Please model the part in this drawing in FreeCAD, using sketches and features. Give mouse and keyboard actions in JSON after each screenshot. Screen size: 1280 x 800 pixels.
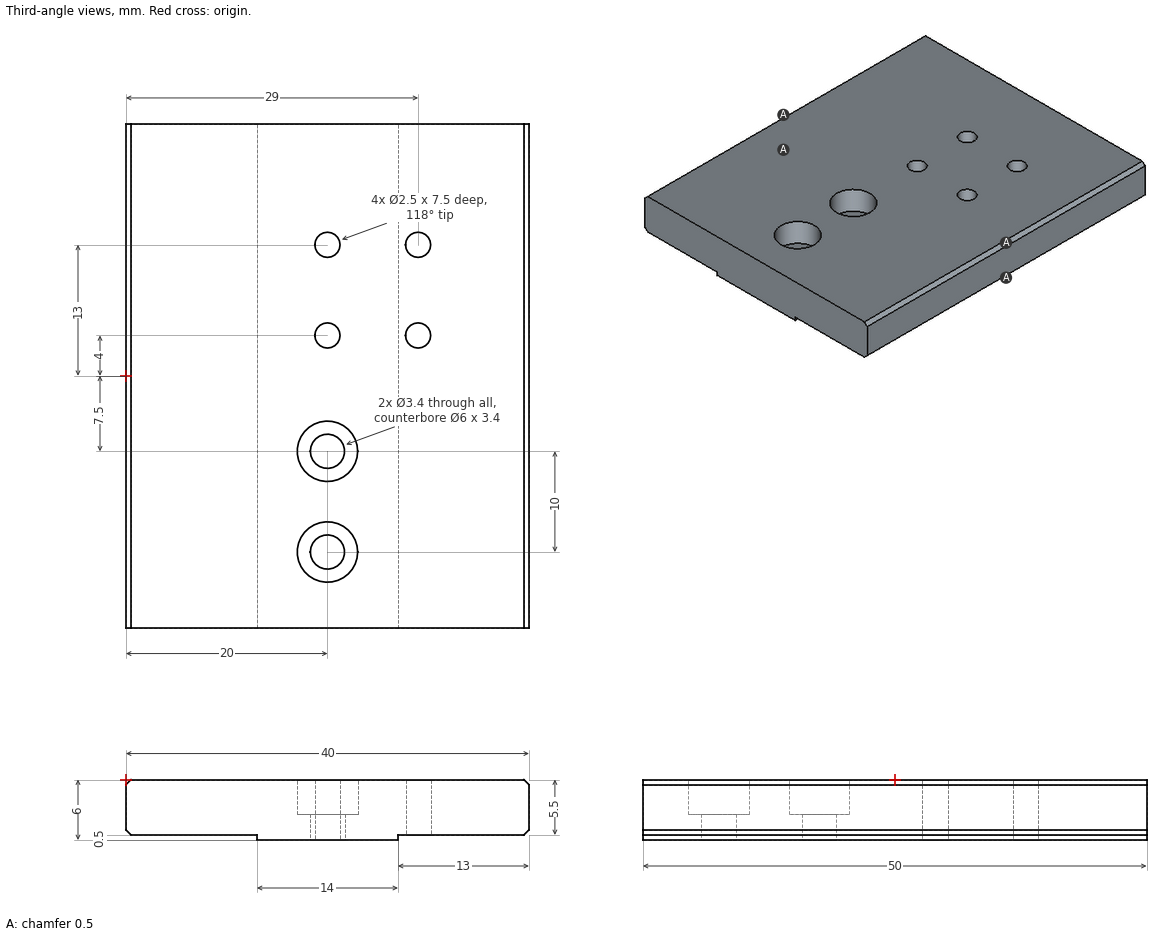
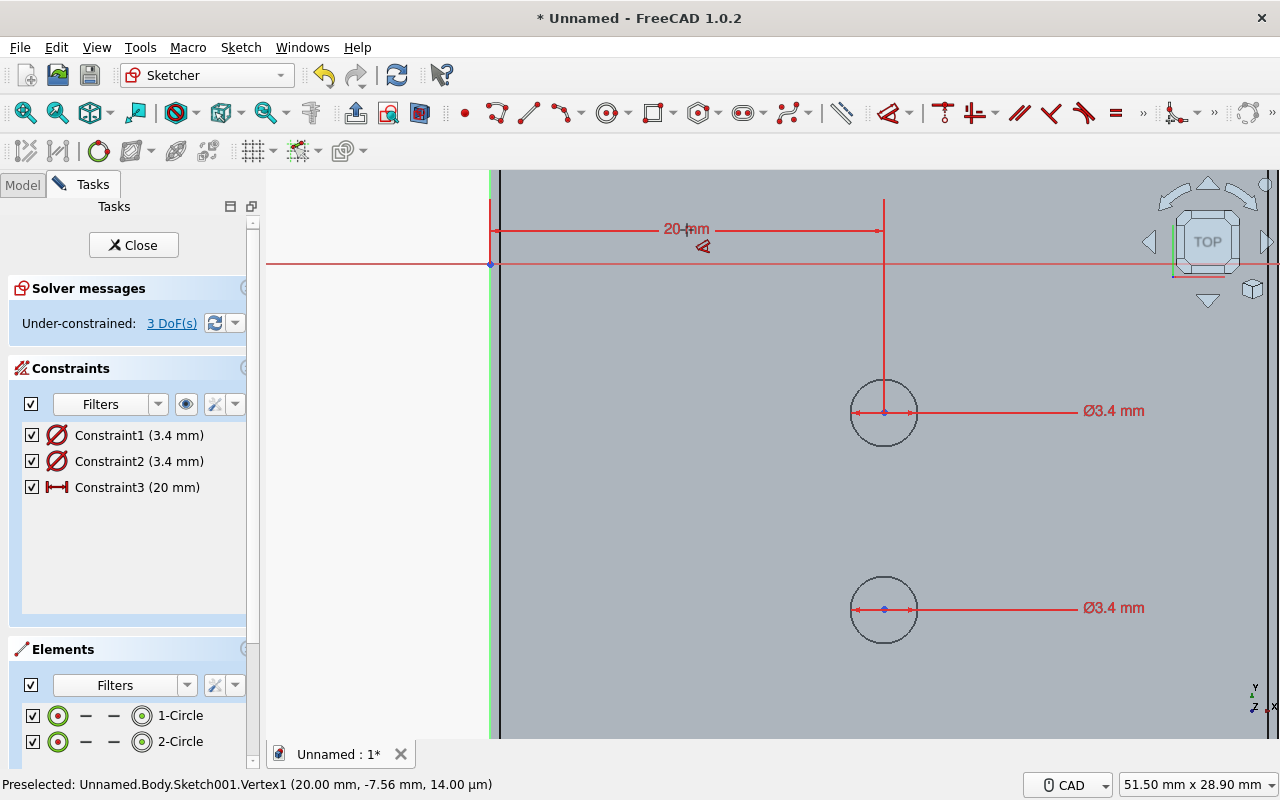
{"action": "left_click", "coordinate": [884, 610]}
{"action": "left_click", "coordinate": [597, 230]}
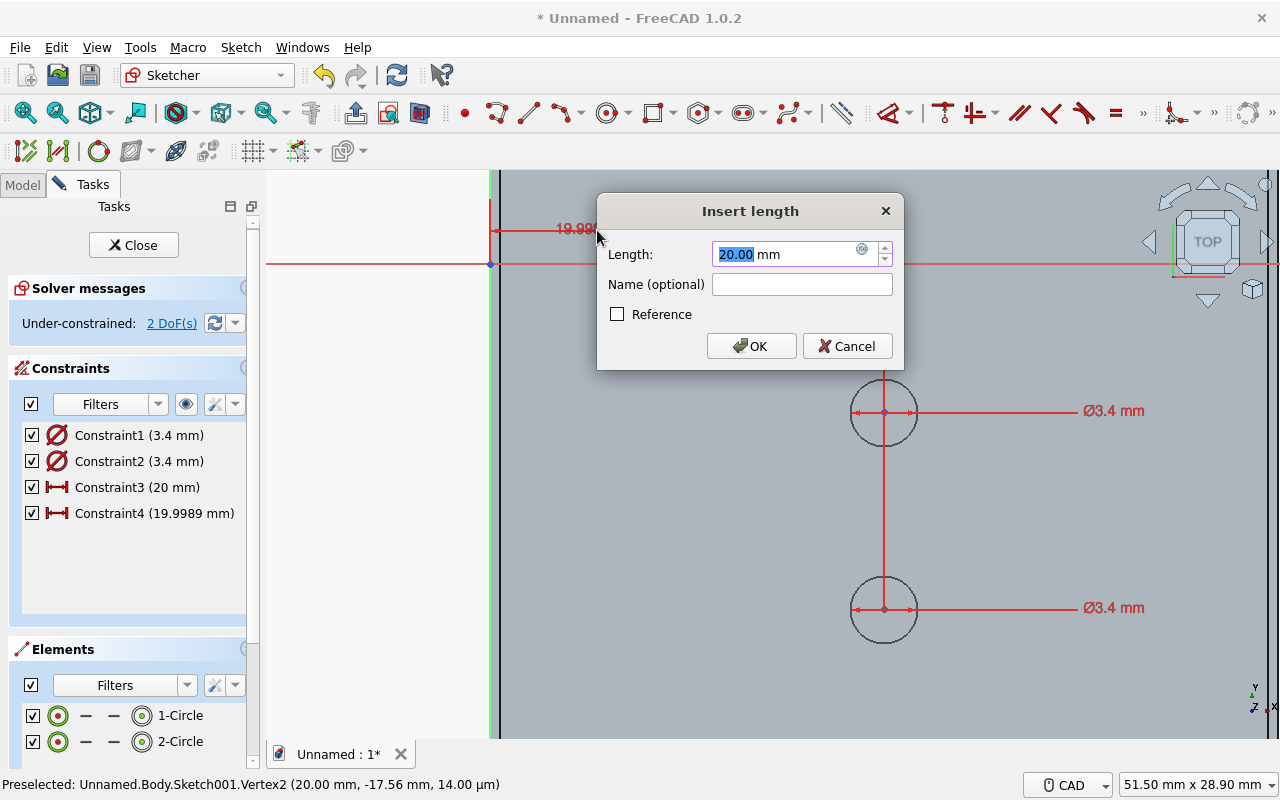
{"action": "type", "text": "20"}
{"action": "key", "text": "Return"}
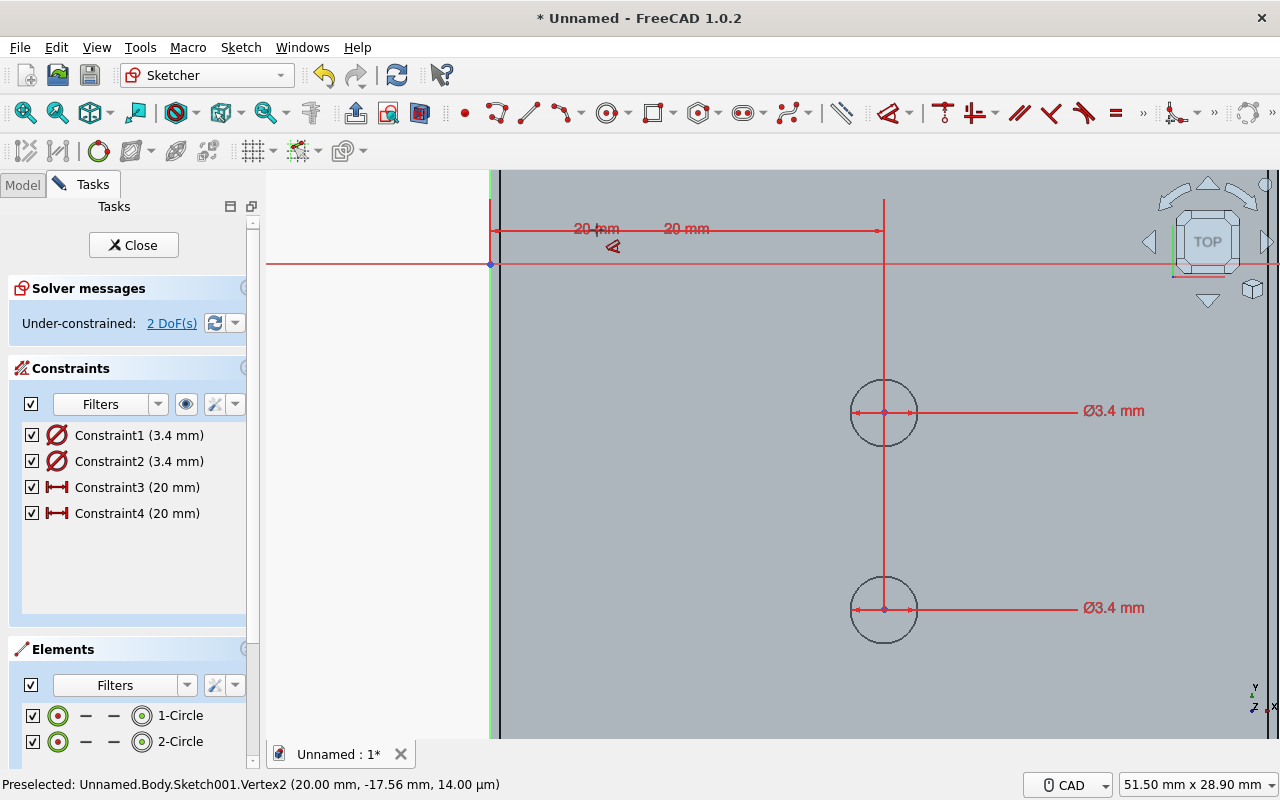
{"action": "left_click", "coordinate": [884, 413]}
{"action": "left_click", "coordinate": [456, 339]}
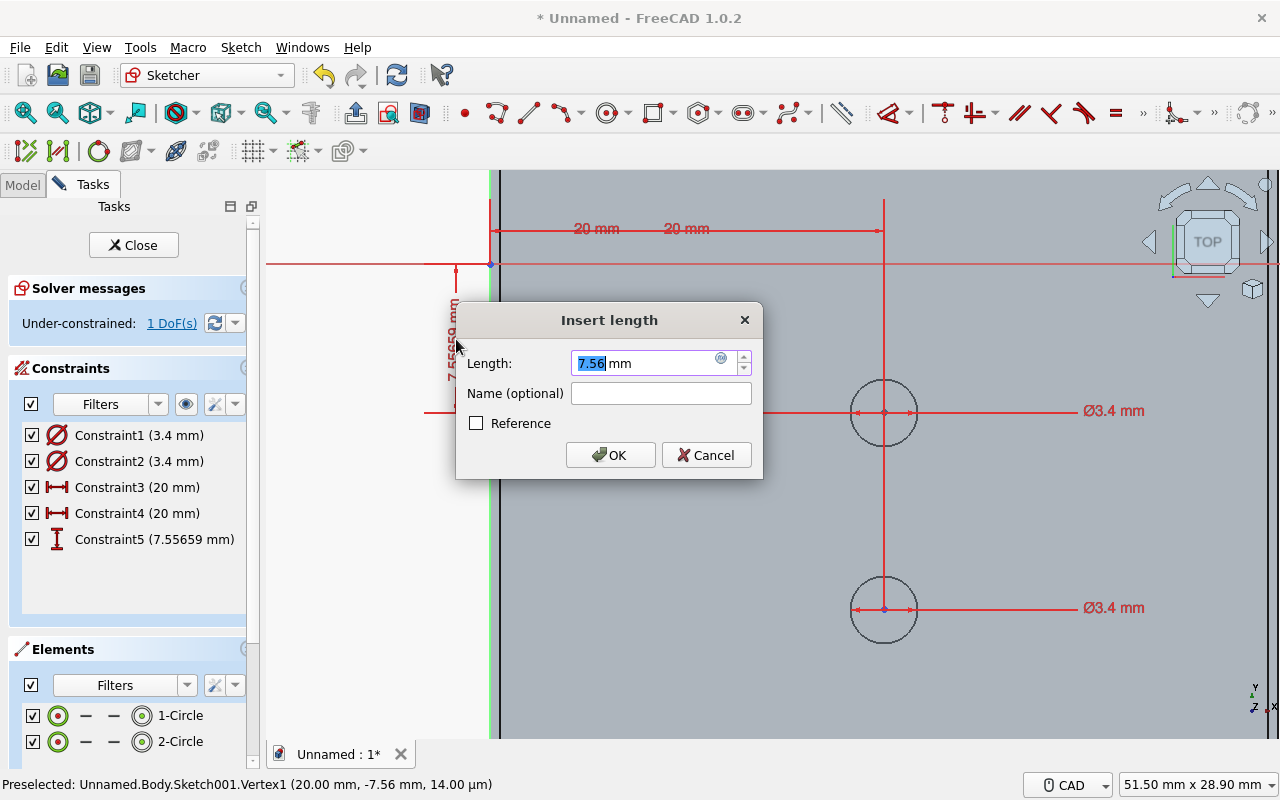
{"action": "type", "text": "7.5"}
{"action": "key", "text": "Return"}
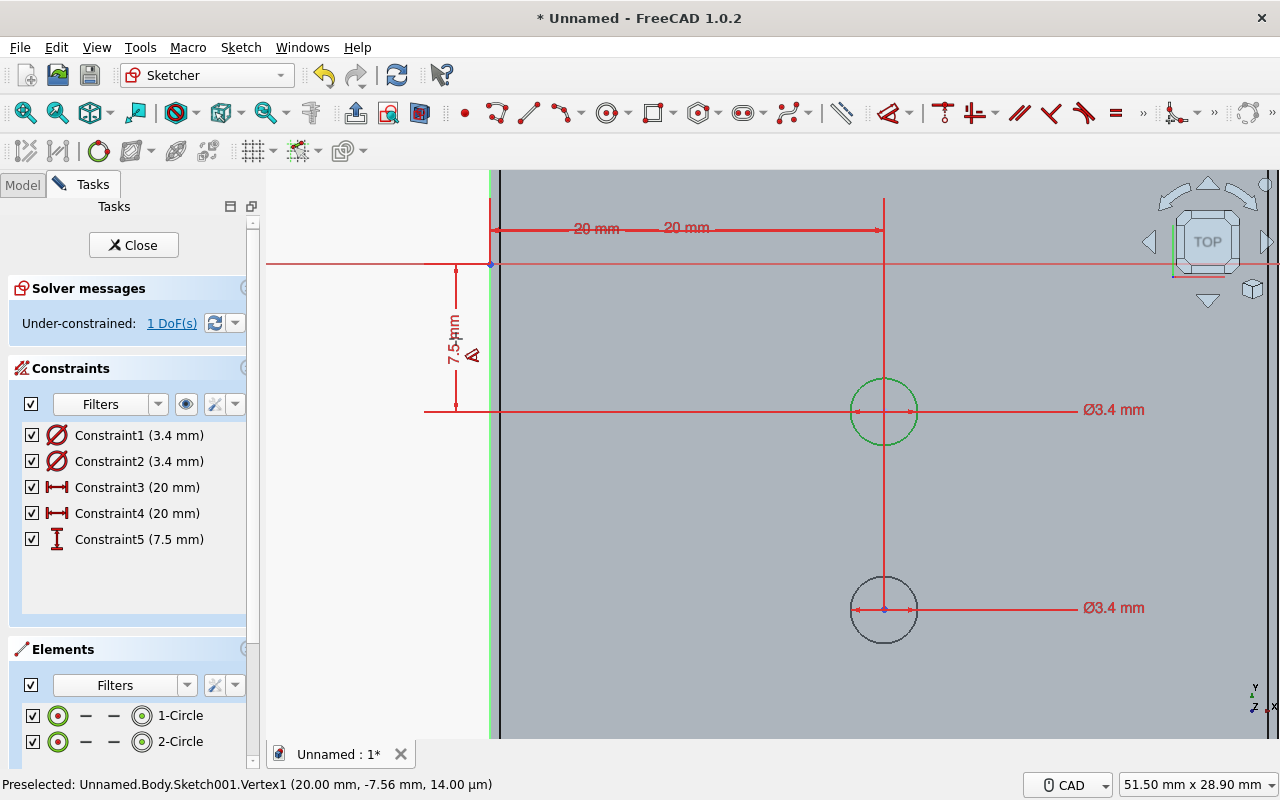
{"action": "left_click", "coordinate": [884, 412]}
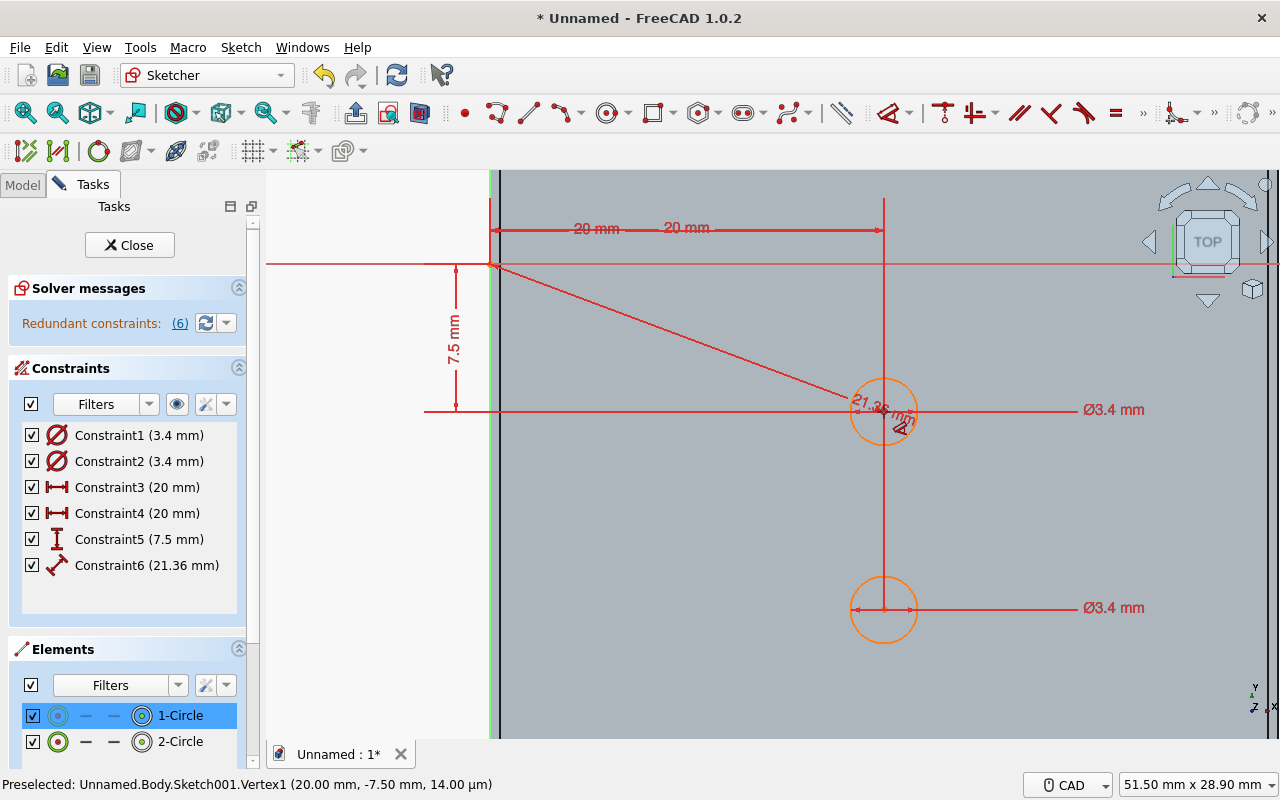
{"action": "left_click", "coordinate": [884, 610]}
{"action": "left_click", "coordinate": [918, 511]}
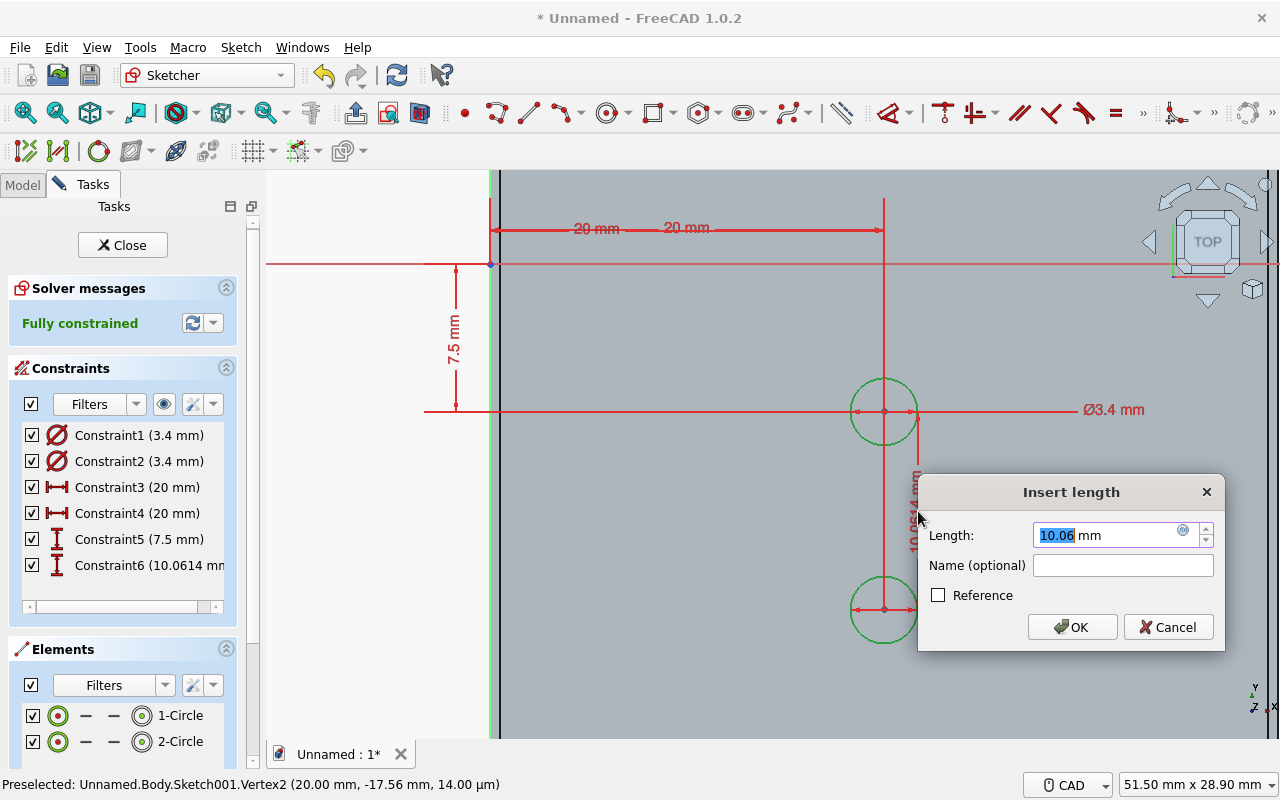
{"action": "type", "text": "10"}
{"action": "key", "text": "Return"}
{"action": "key", "text": "Escape"}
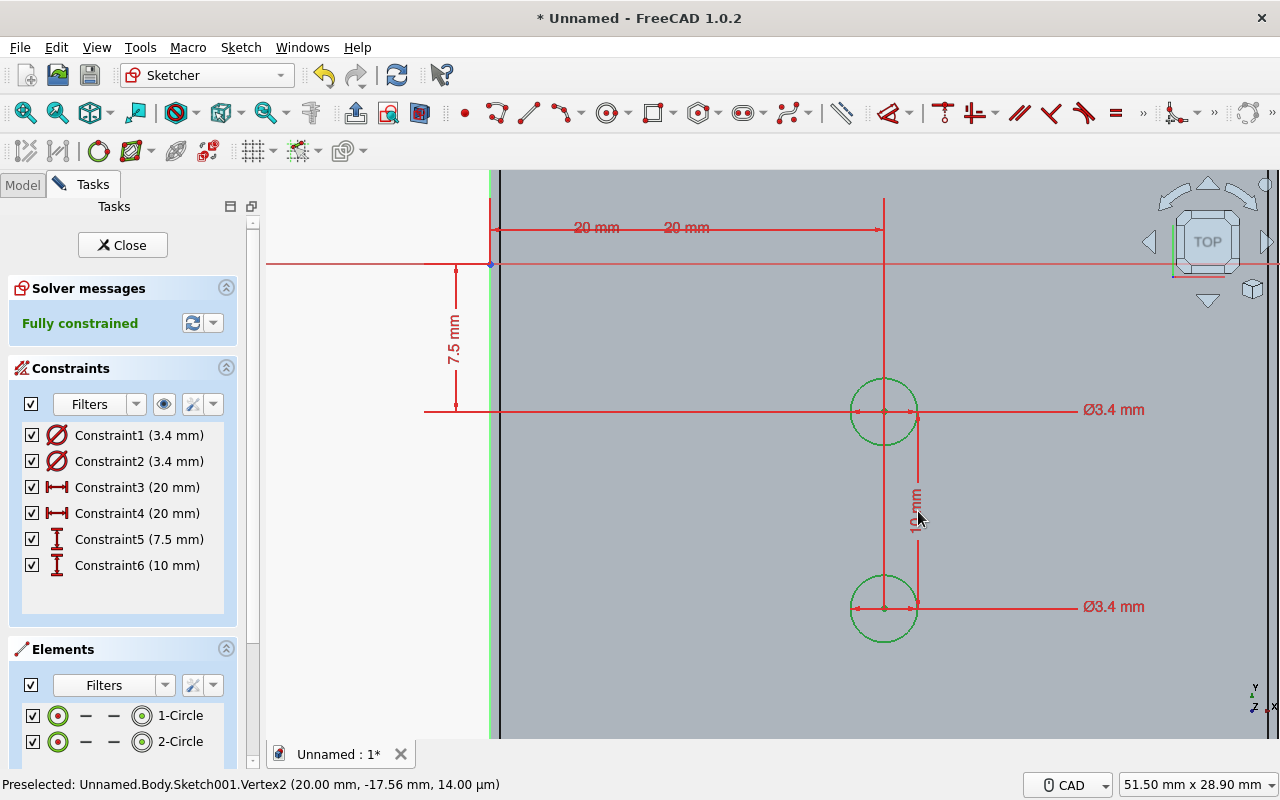
{"action": "left_click", "coordinate": [123, 245]}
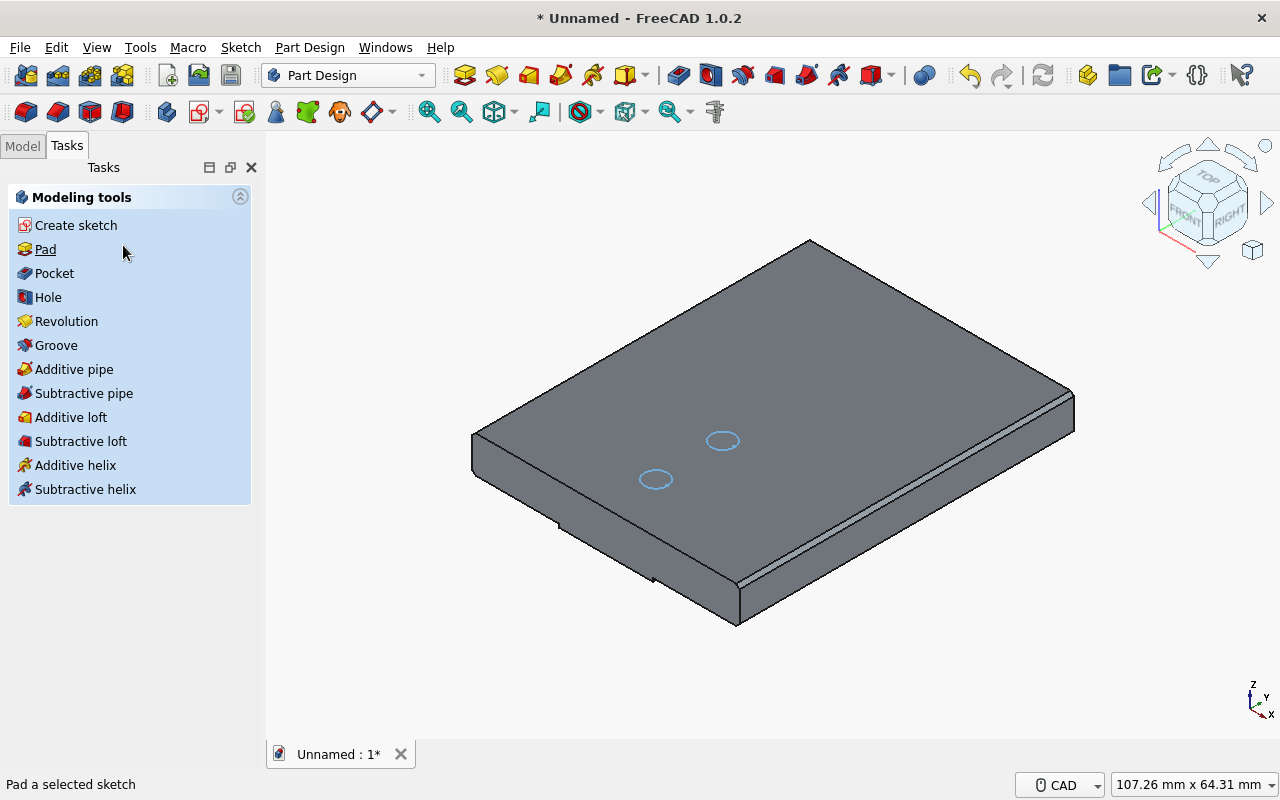
{"action": "left_click", "coordinate": [712, 76]}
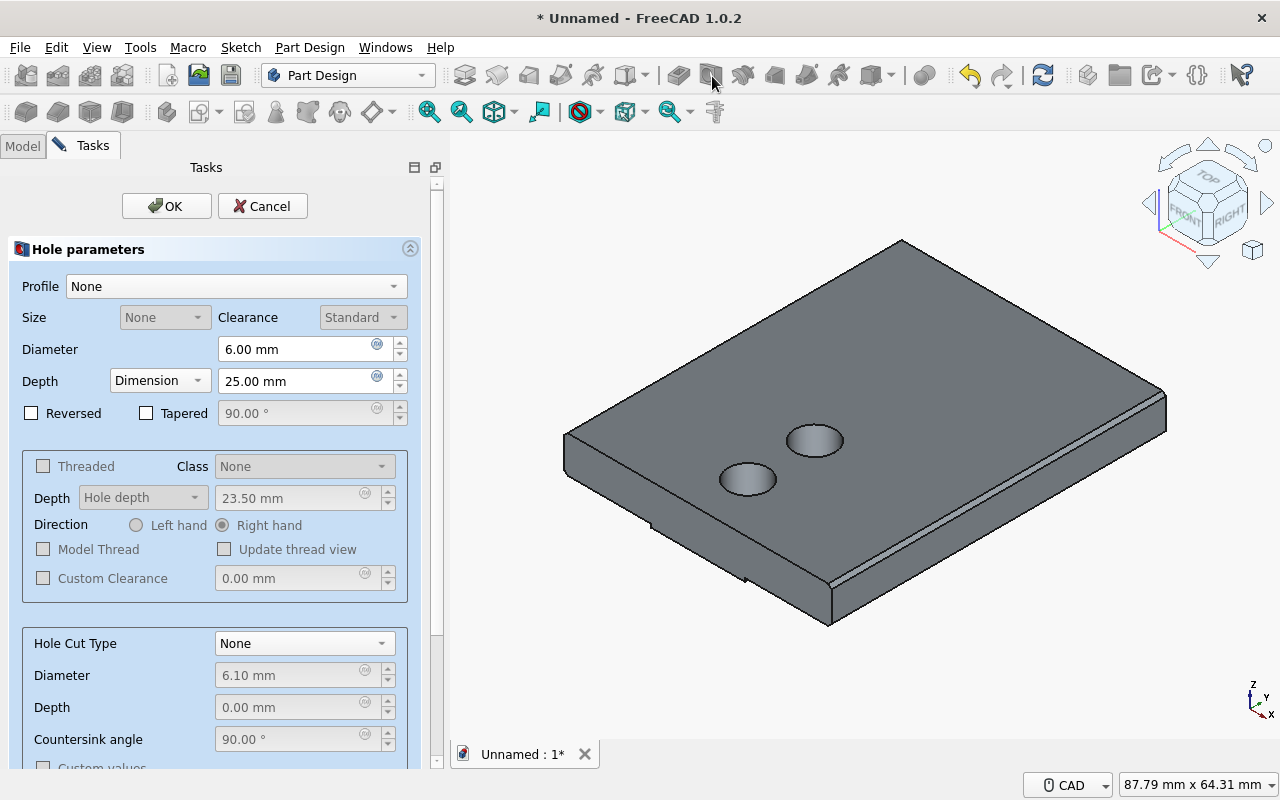
{"action": "triple_click", "coordinate": [305, 349]}